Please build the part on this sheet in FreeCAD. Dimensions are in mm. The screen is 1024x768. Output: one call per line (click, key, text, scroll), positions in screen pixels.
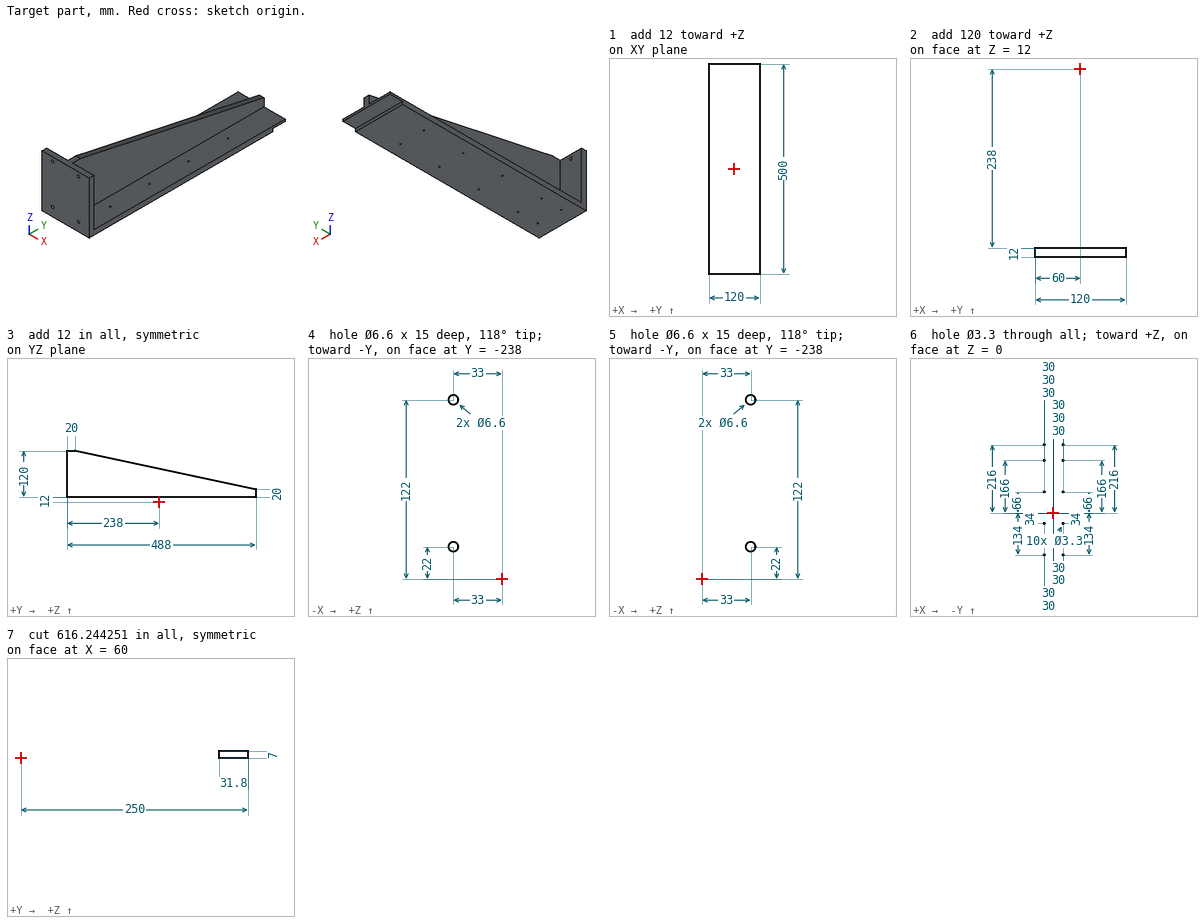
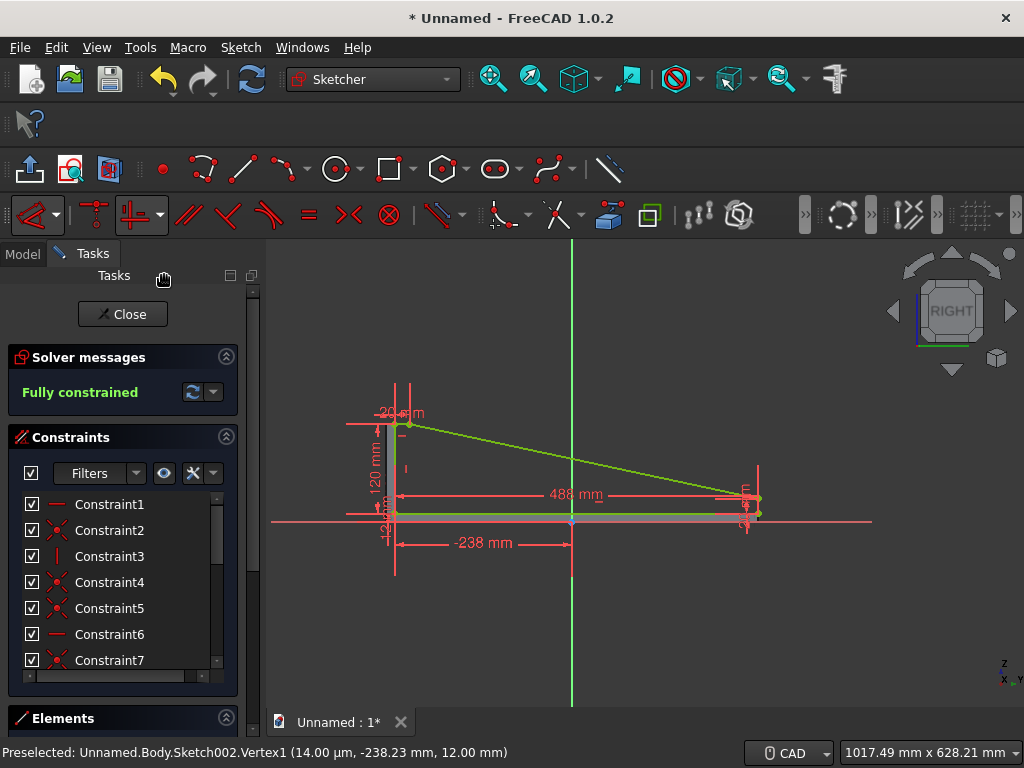
click(123, 314)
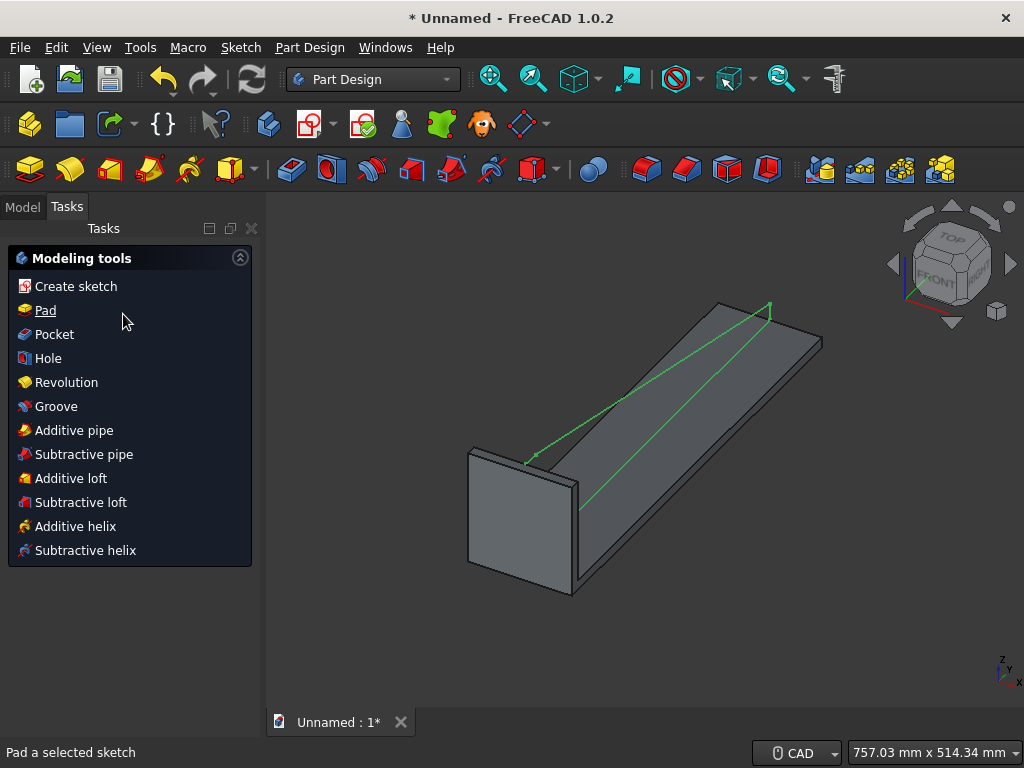
click(30, 170)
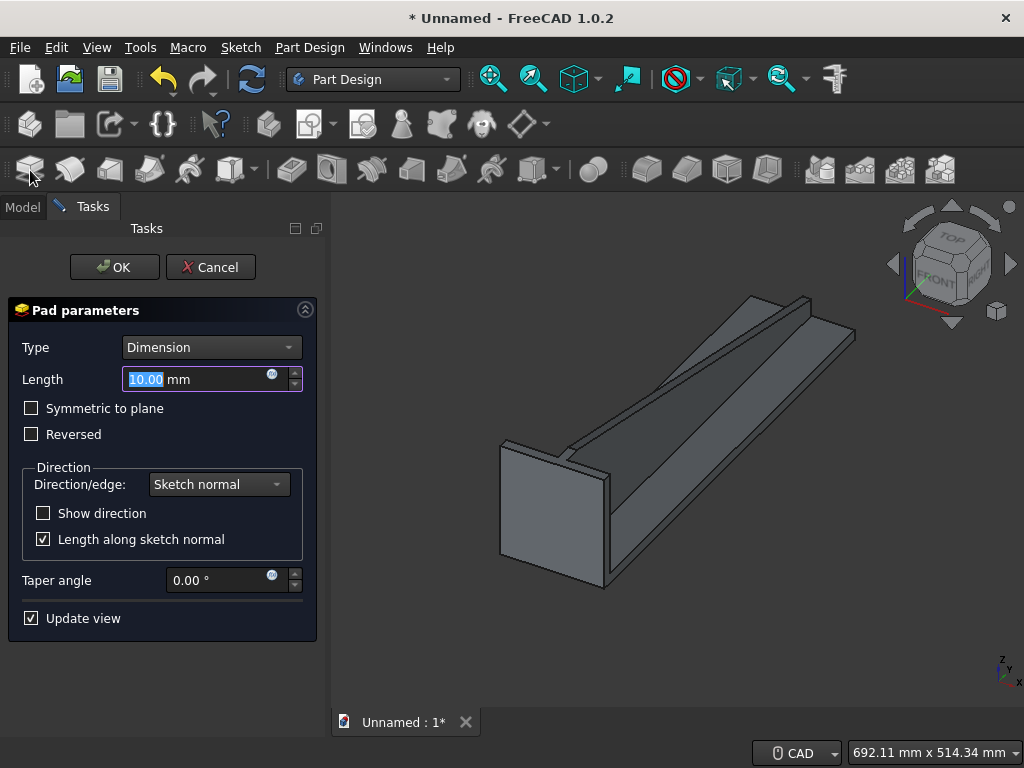
text(12)
key(Tab)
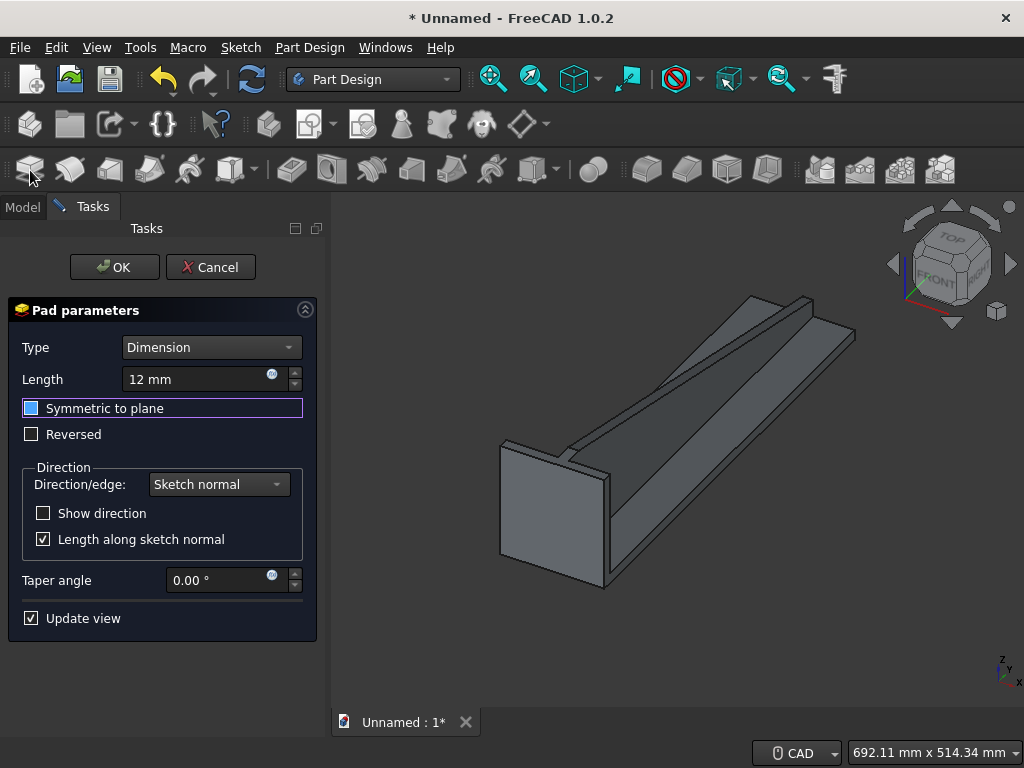
click(30, 408)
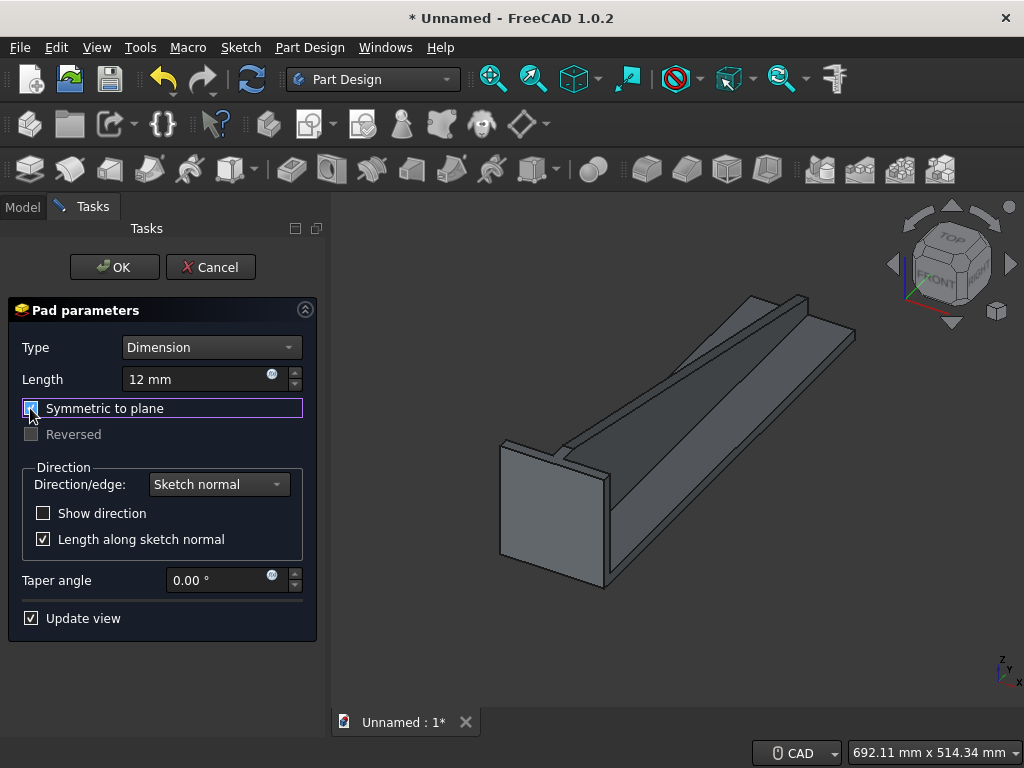
click(115, 267)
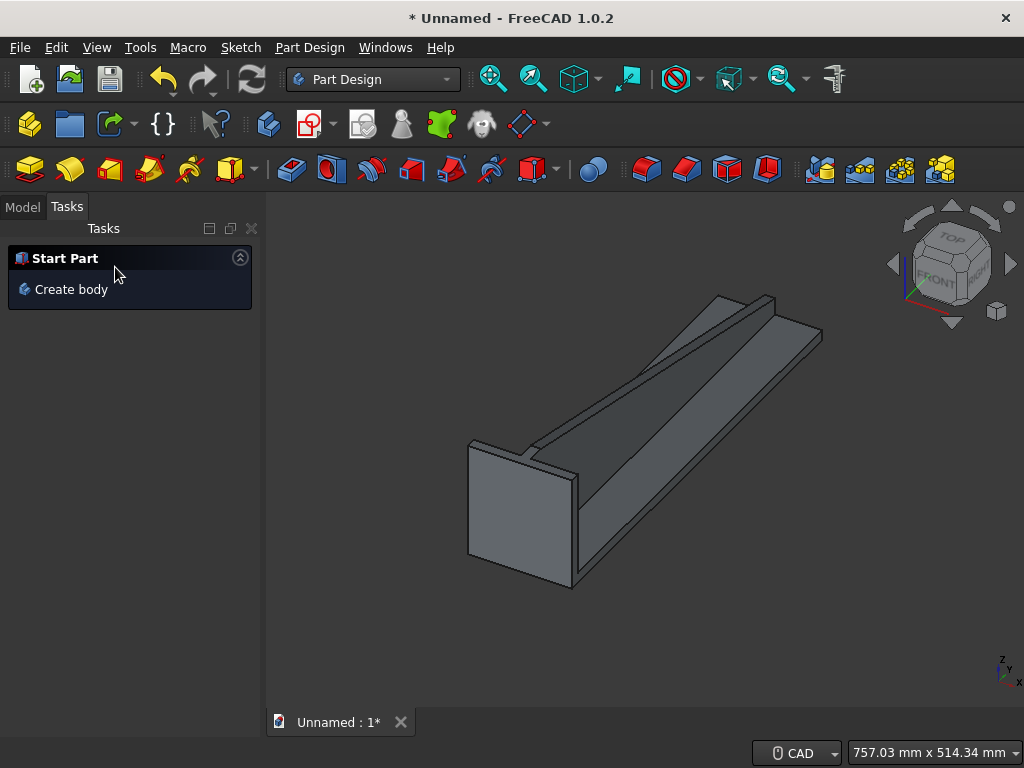
key(4)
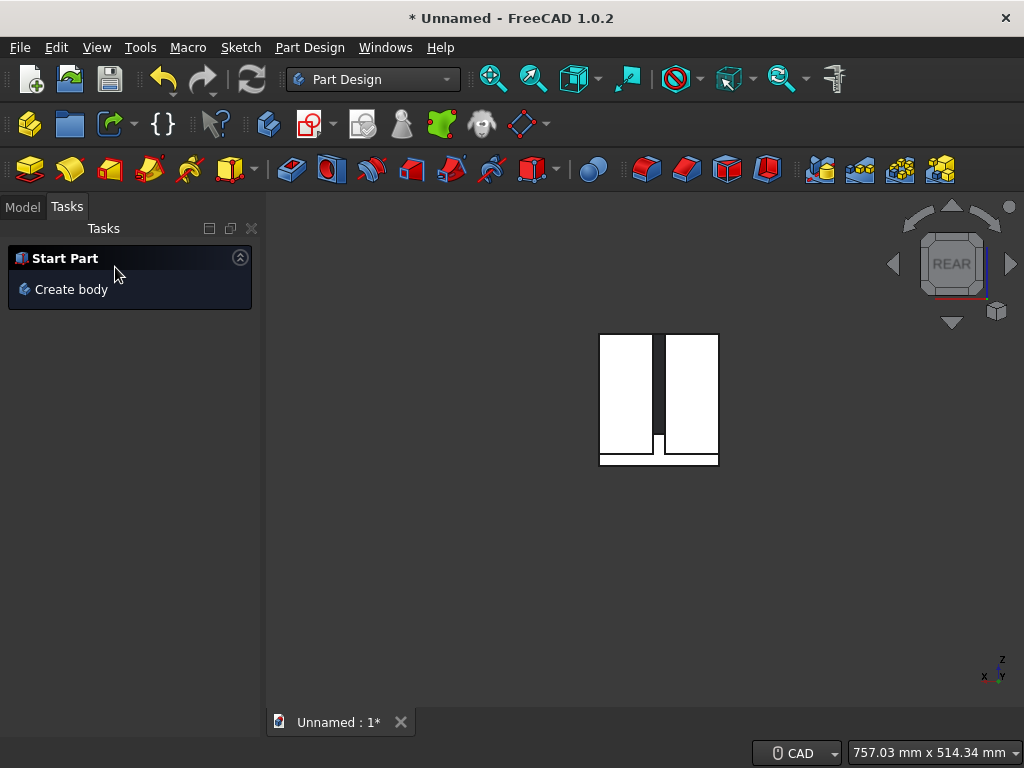
click(494, 80)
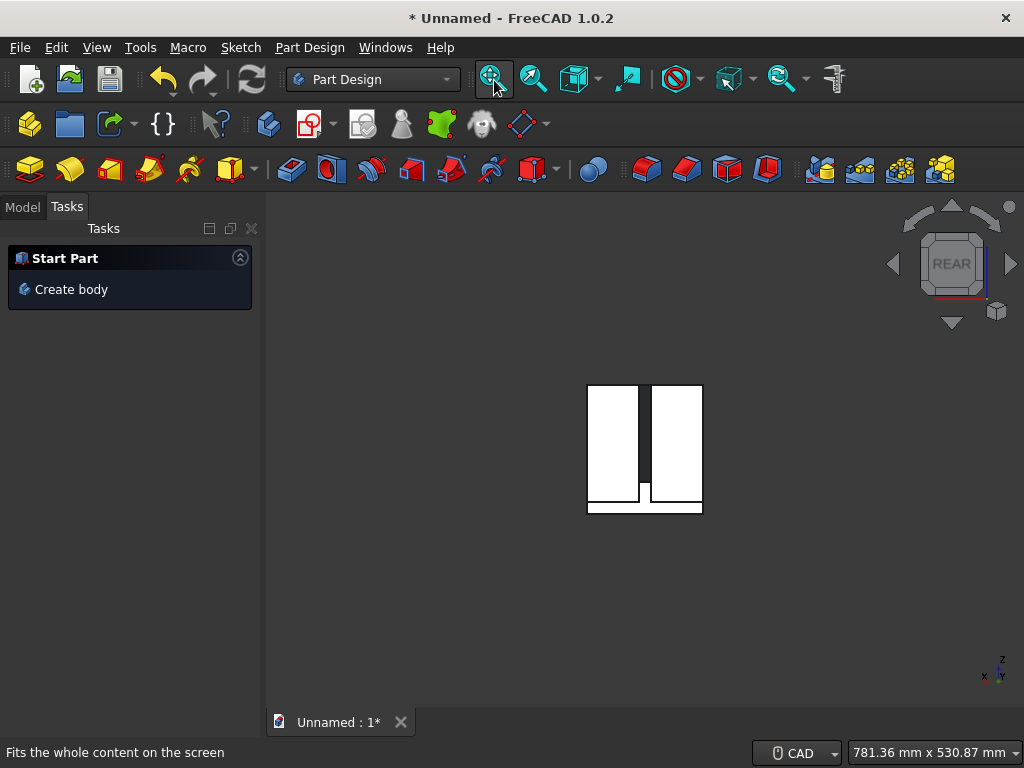
click(677, 426)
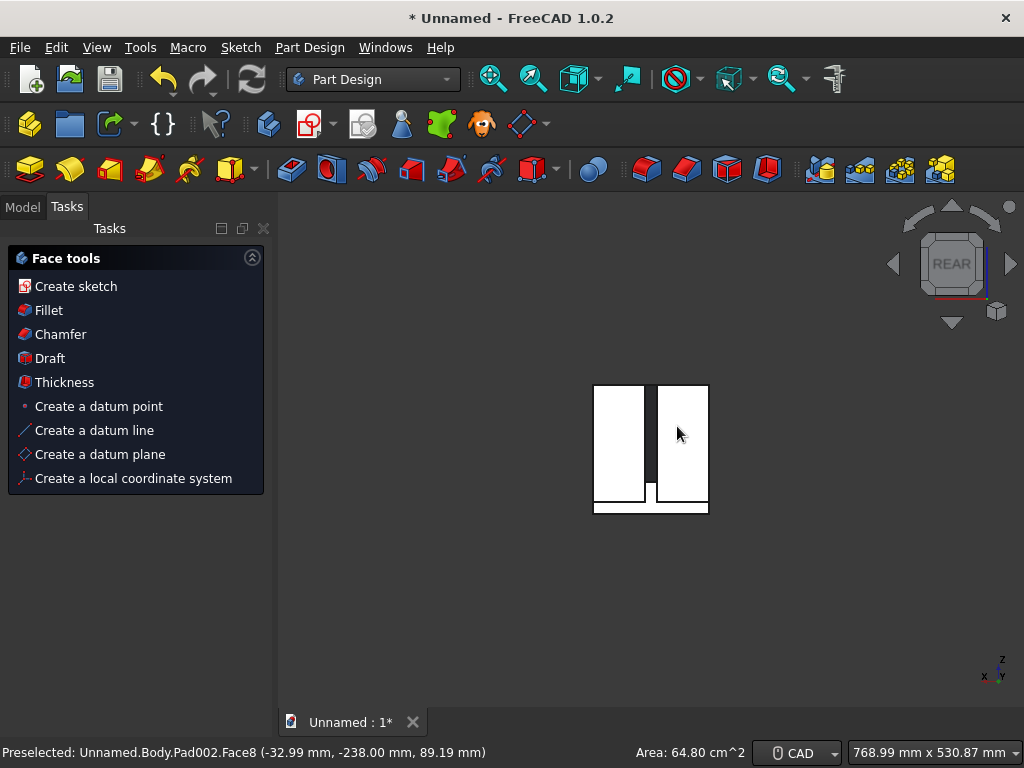
click(310, 124)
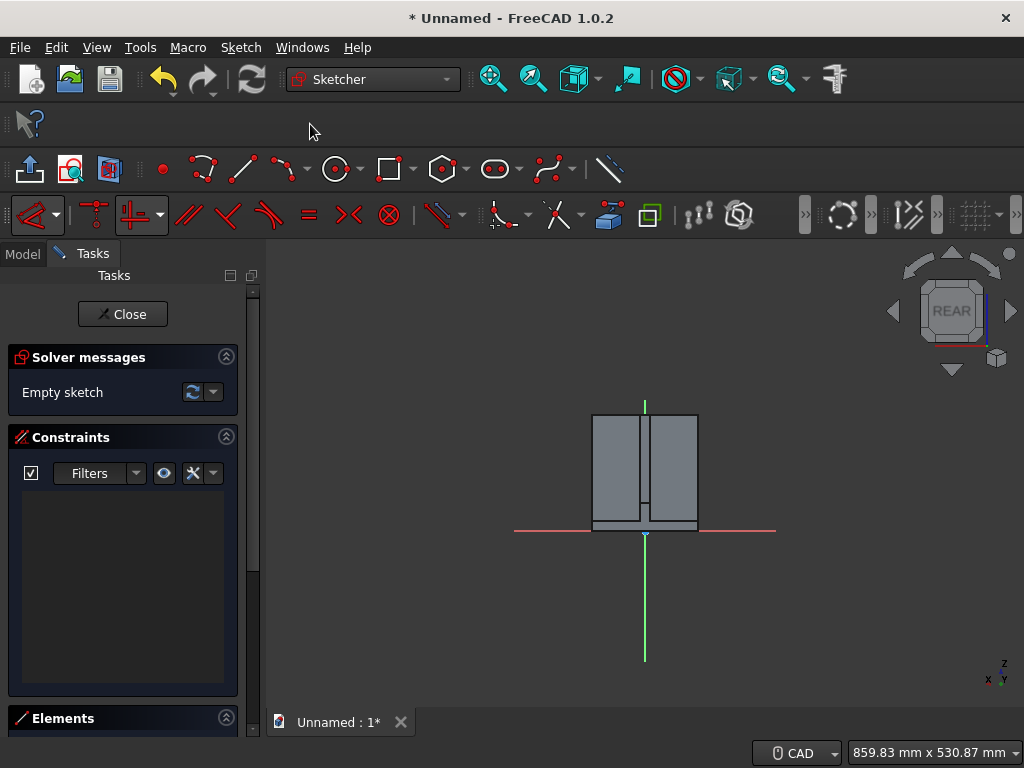
click(110, 170)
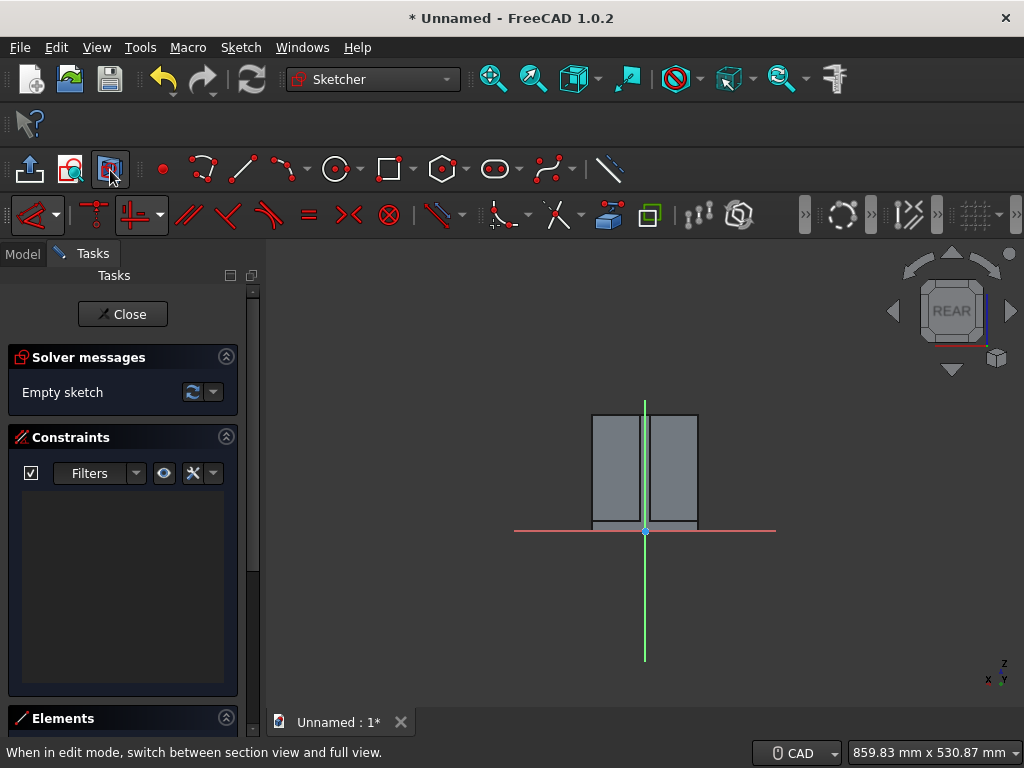
scroll(660, 478, up, 5)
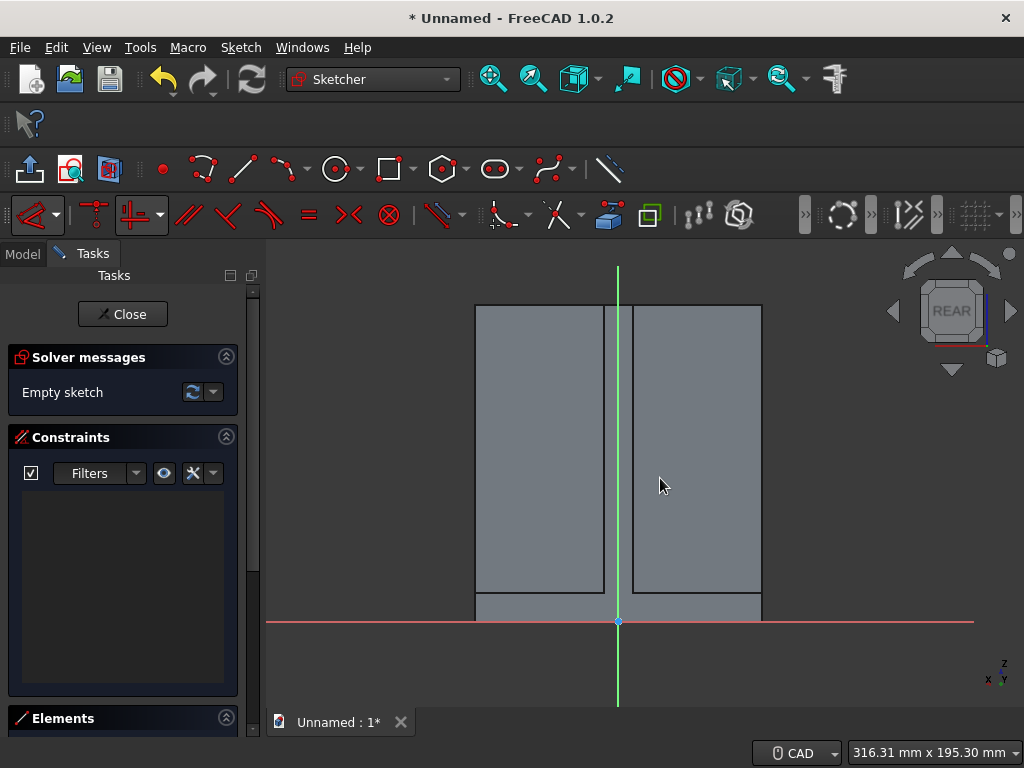
click(336, 170)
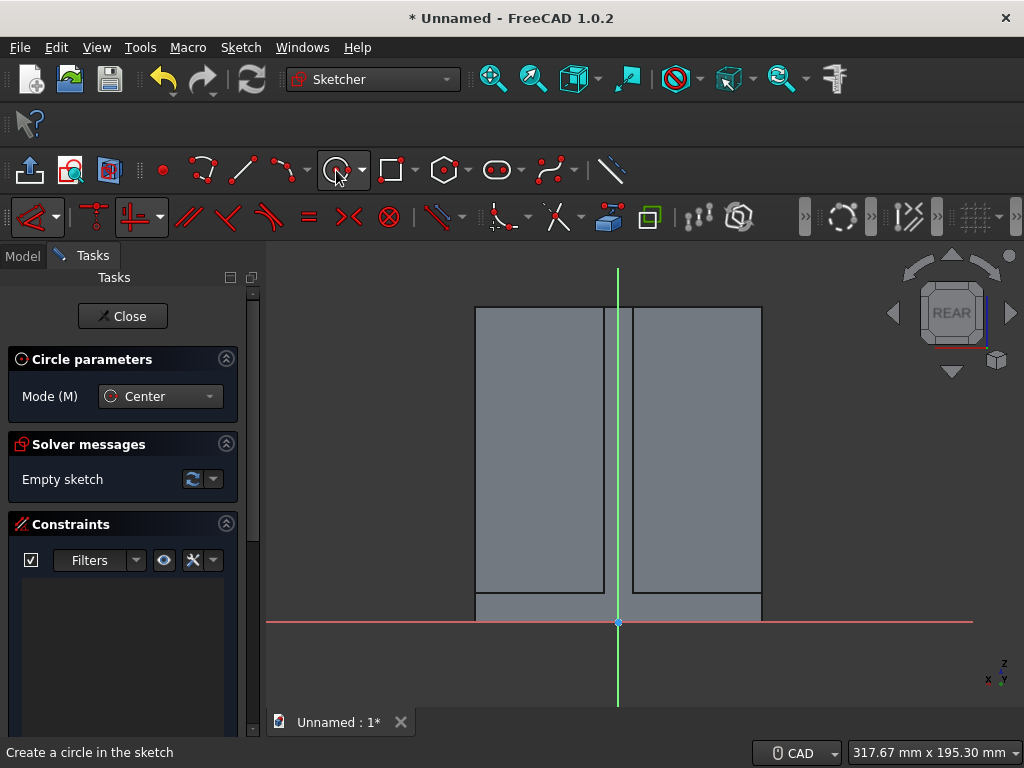
scroll(540, 331, up, 6)